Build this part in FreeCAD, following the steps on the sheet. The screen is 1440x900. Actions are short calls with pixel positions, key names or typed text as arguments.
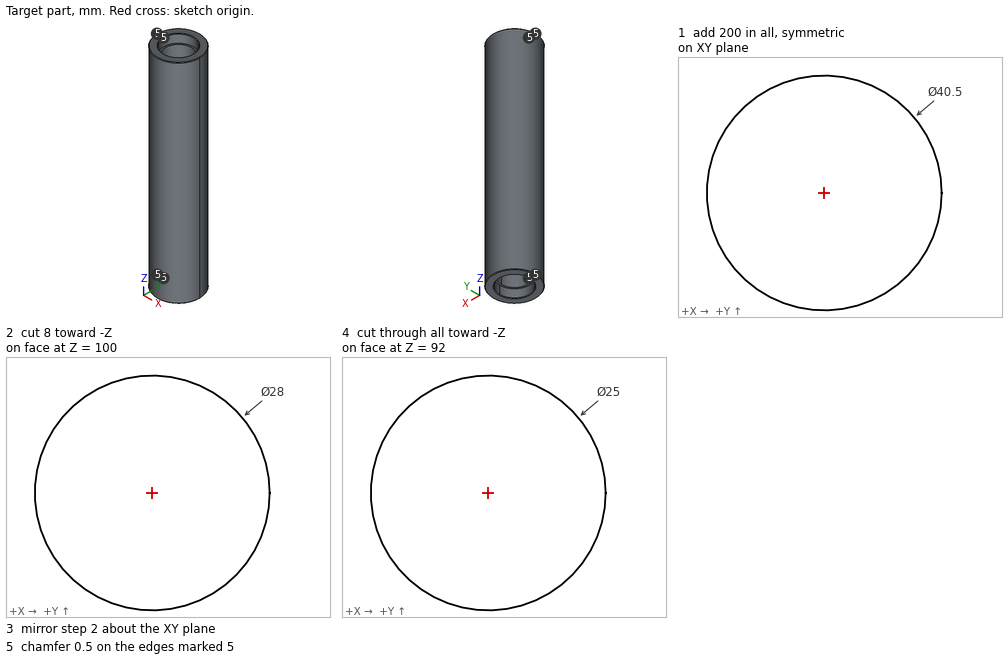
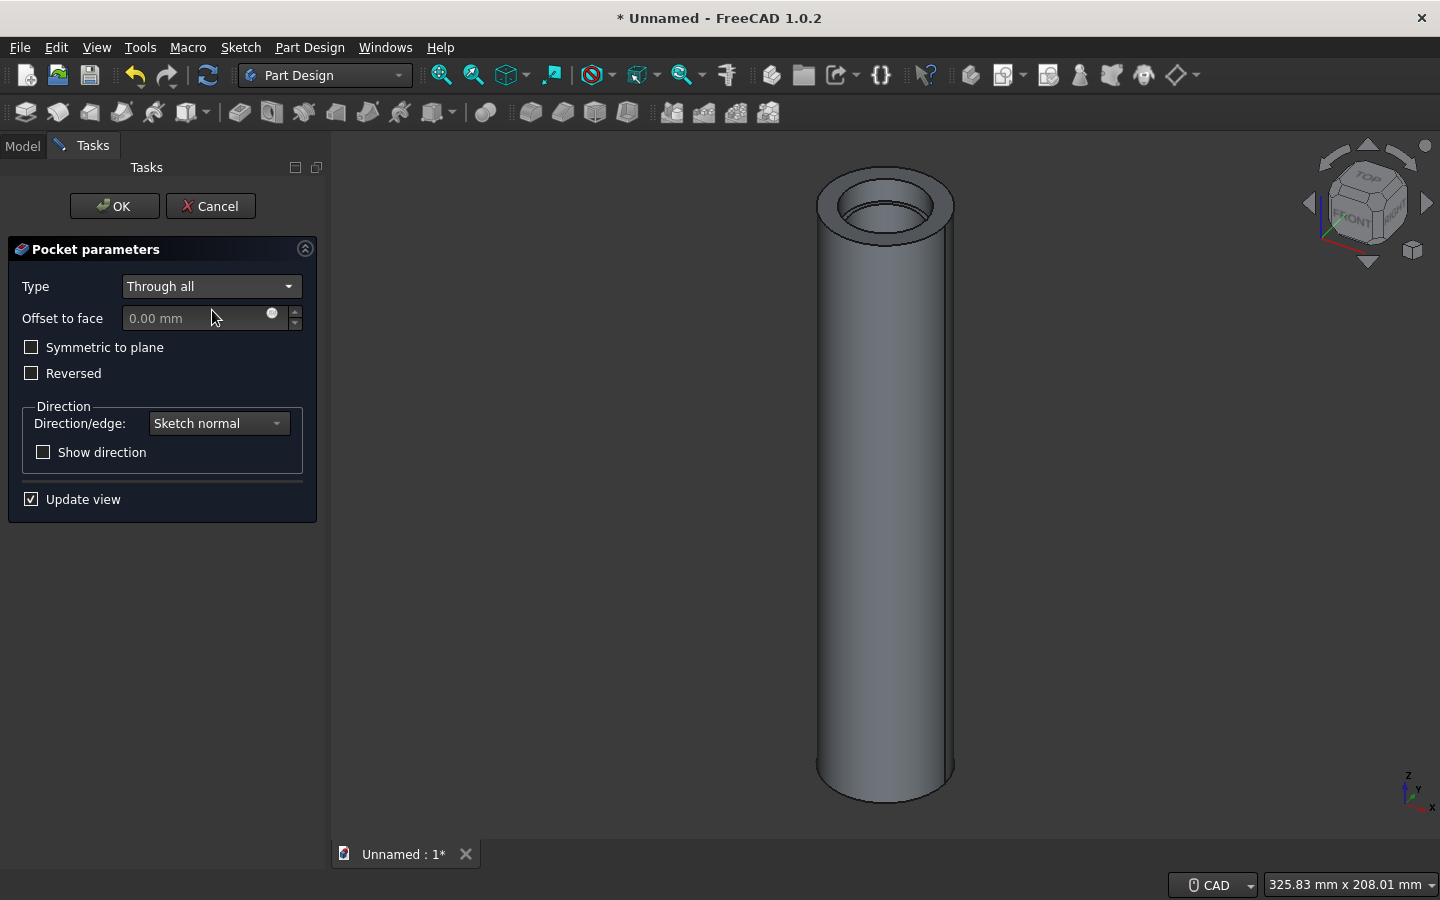
click(115, 206)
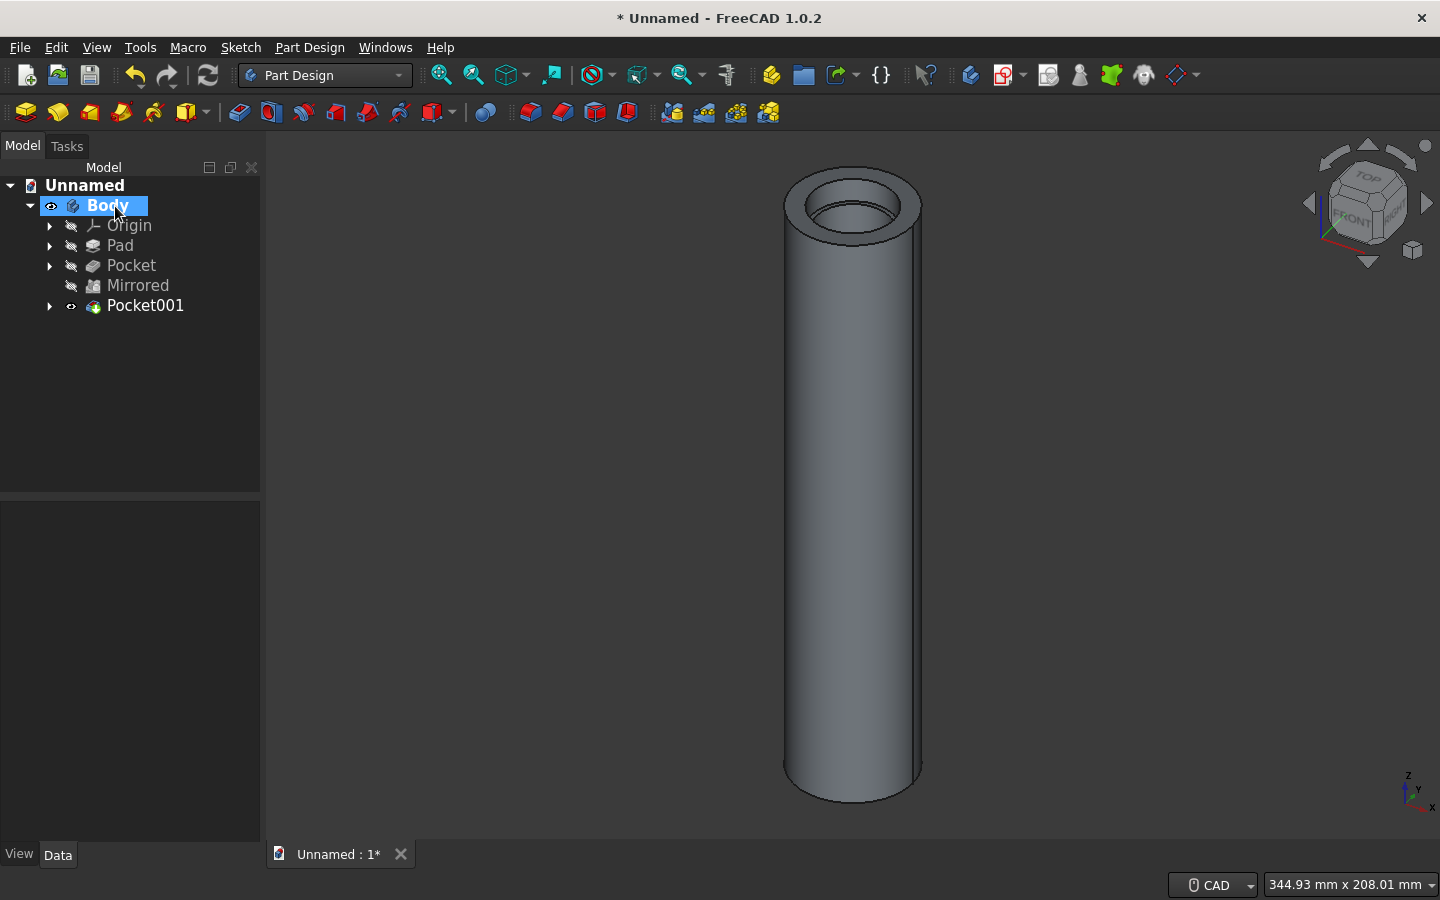
click(784, 209)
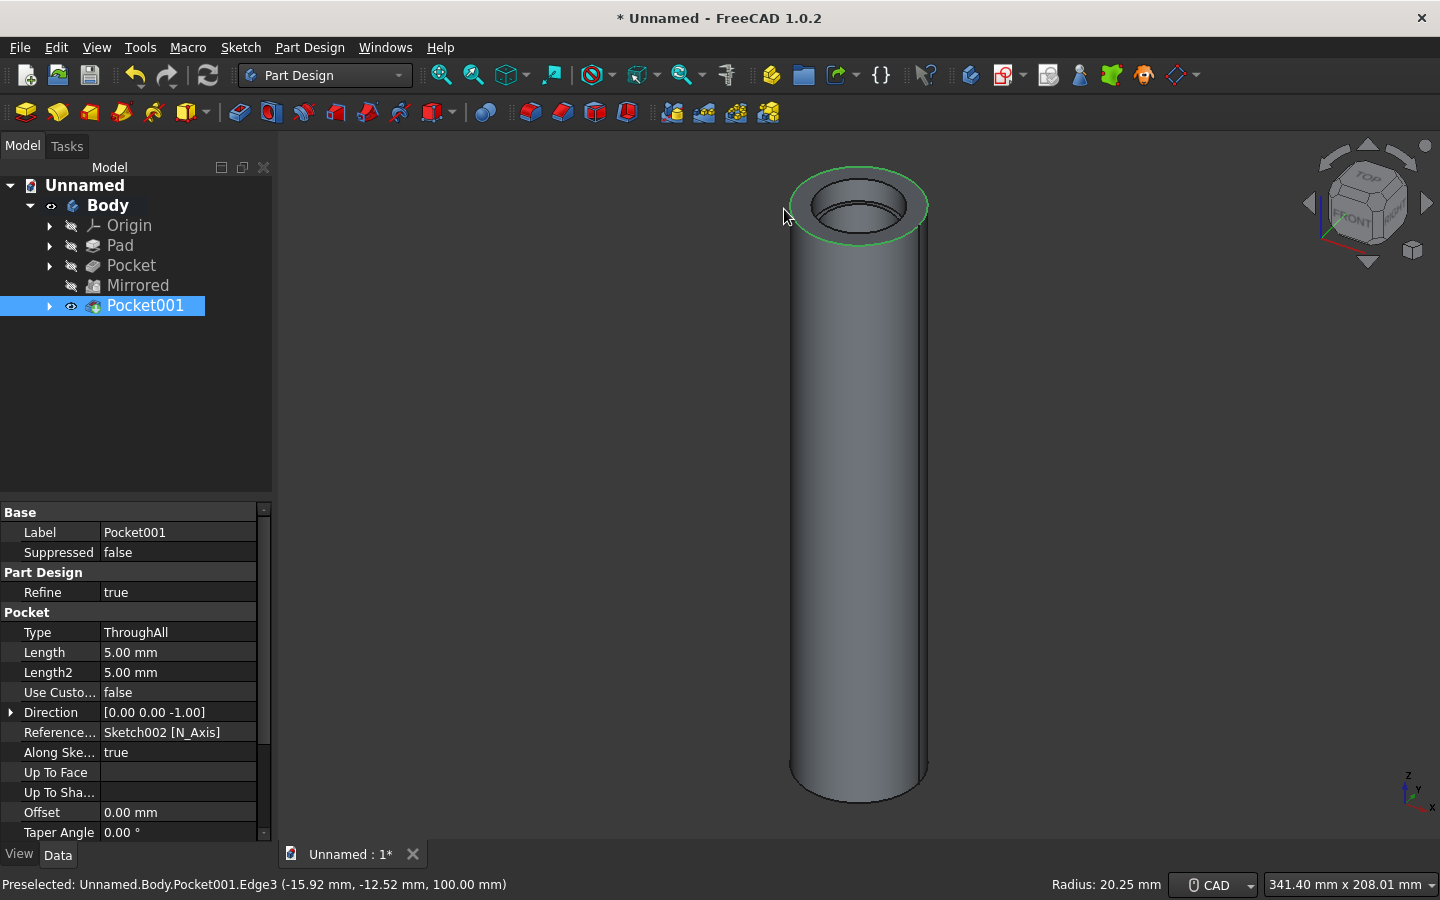
click(818, 191, ctrl)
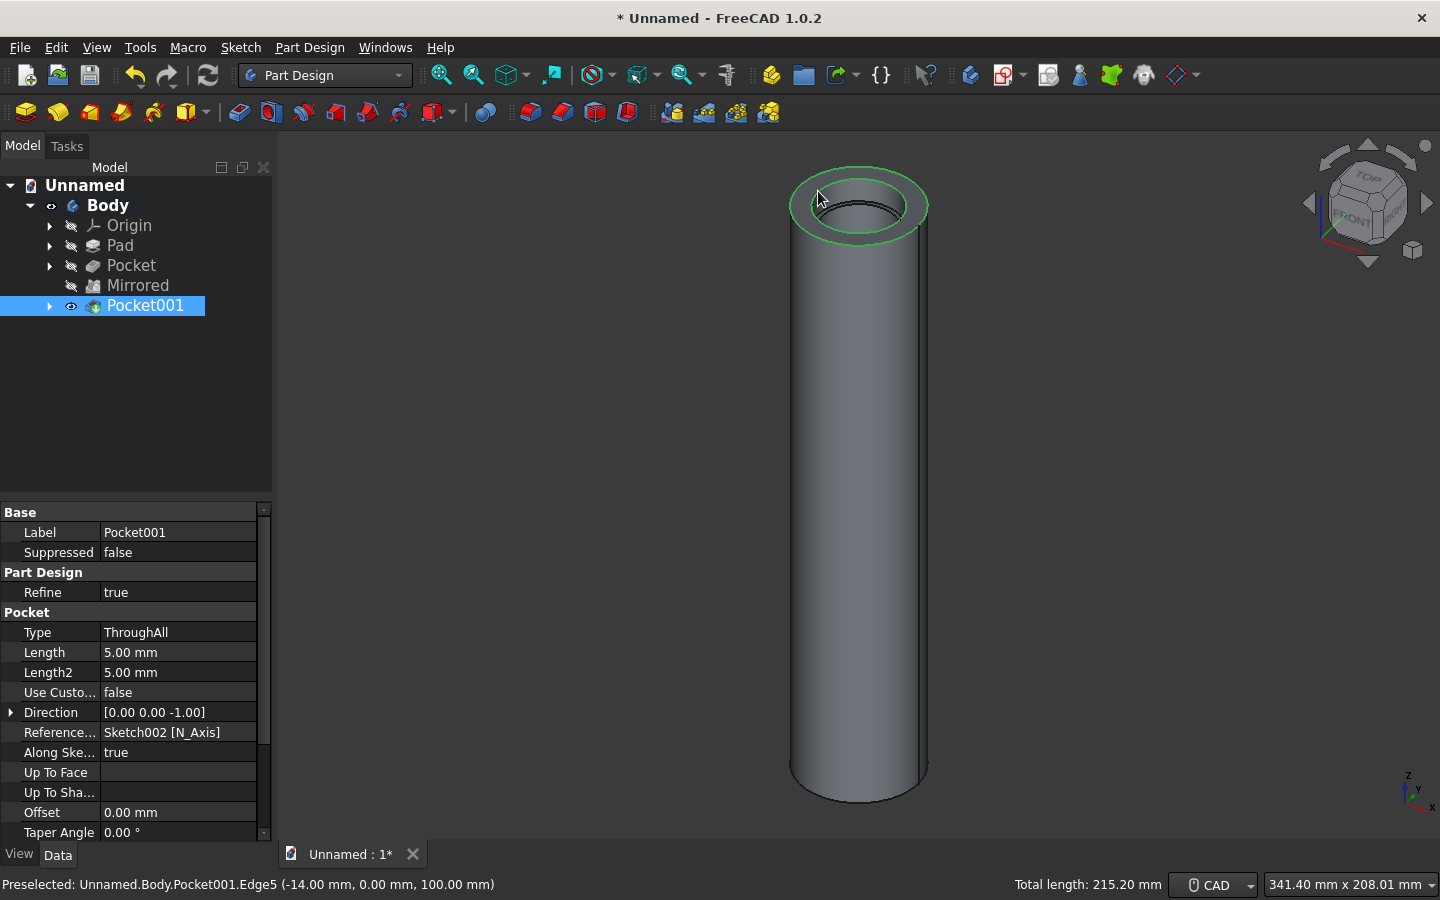
key(0)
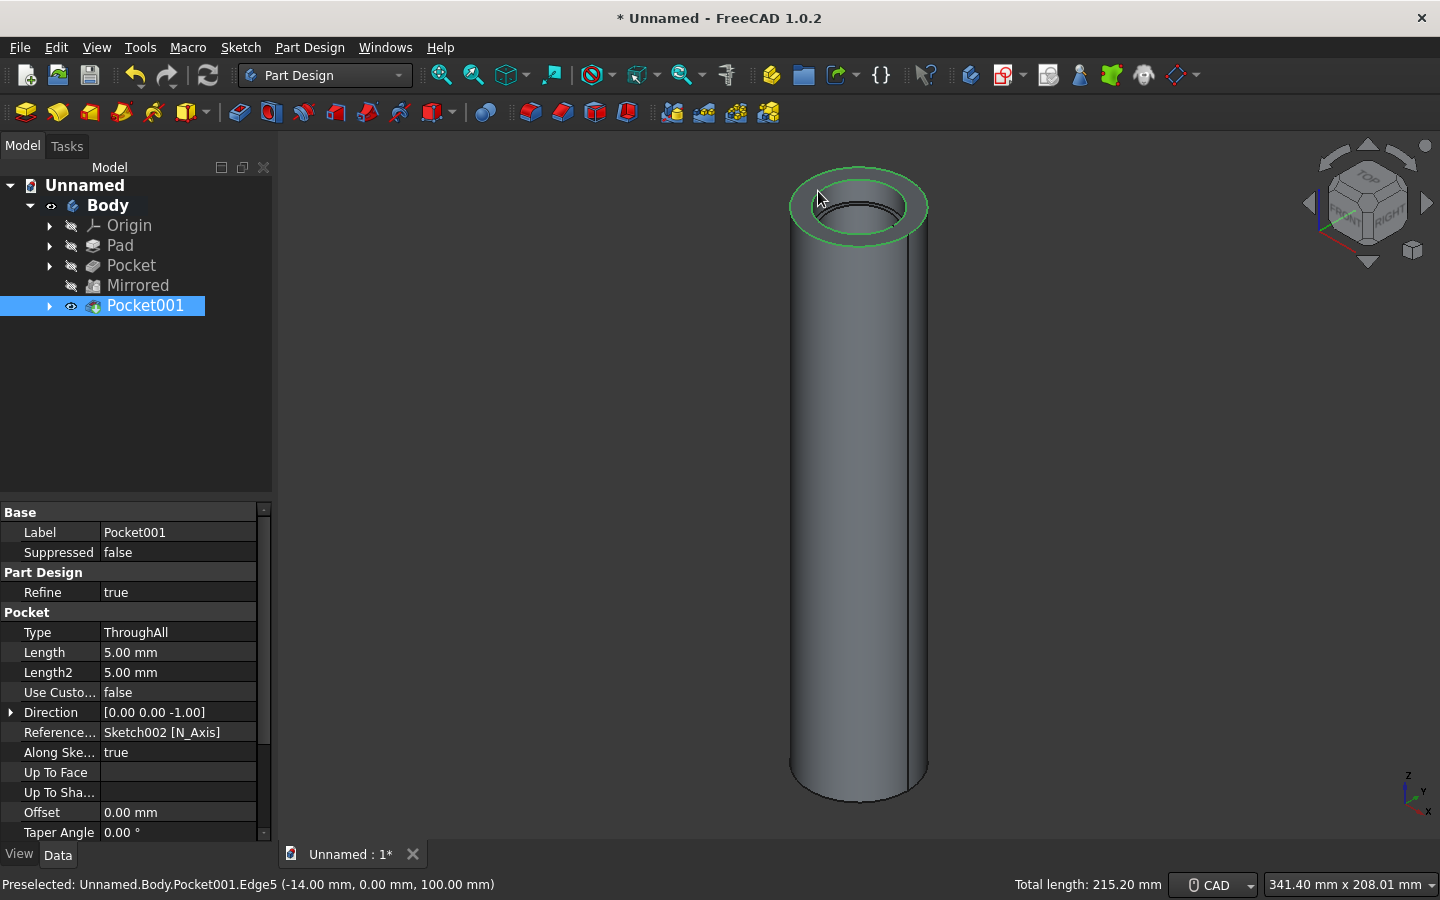
key(2)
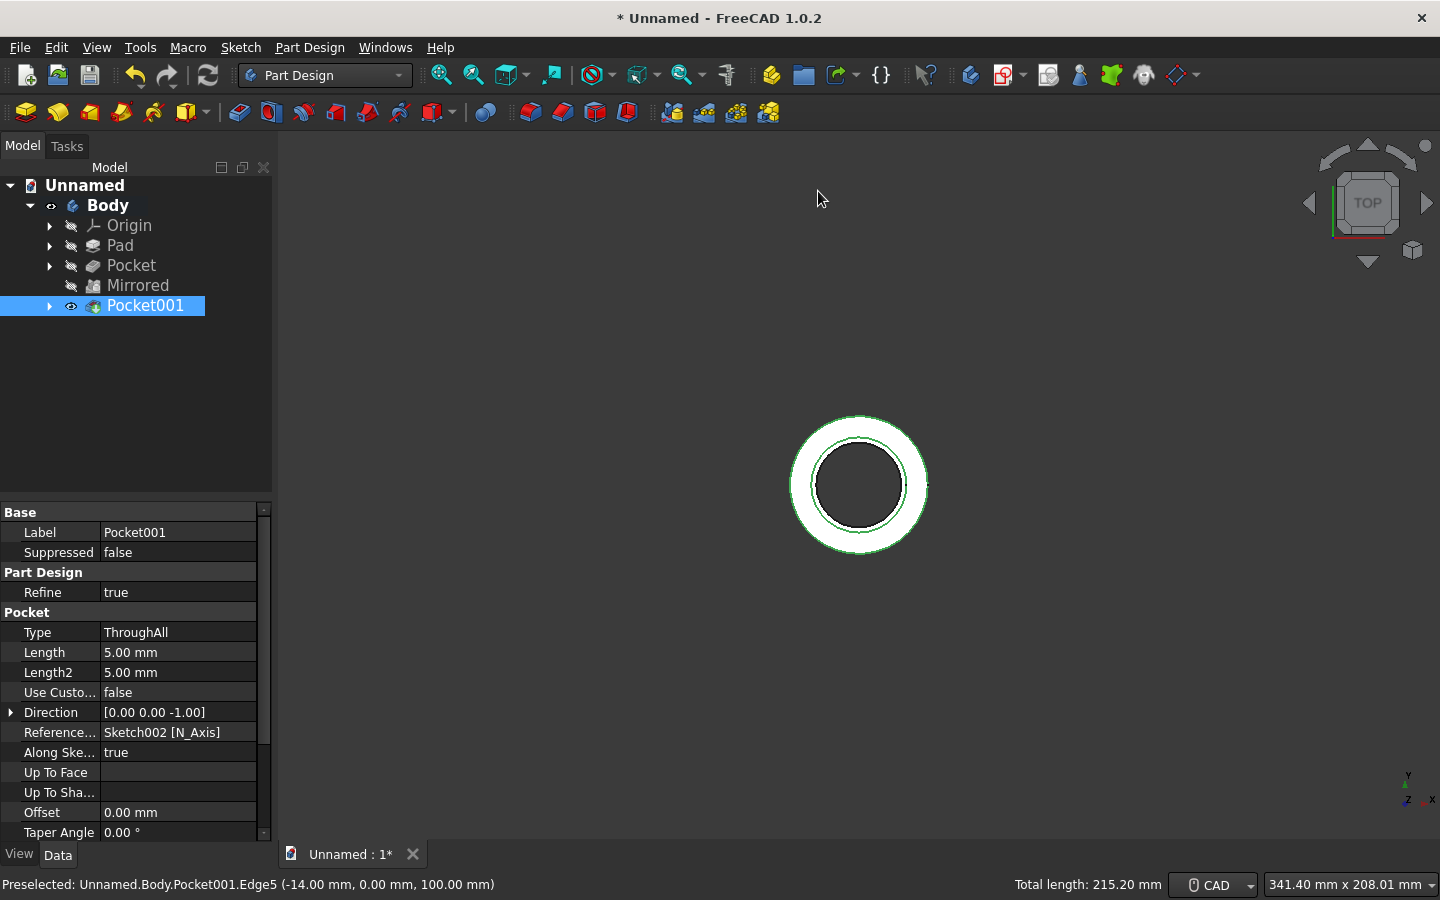
click(442, 76)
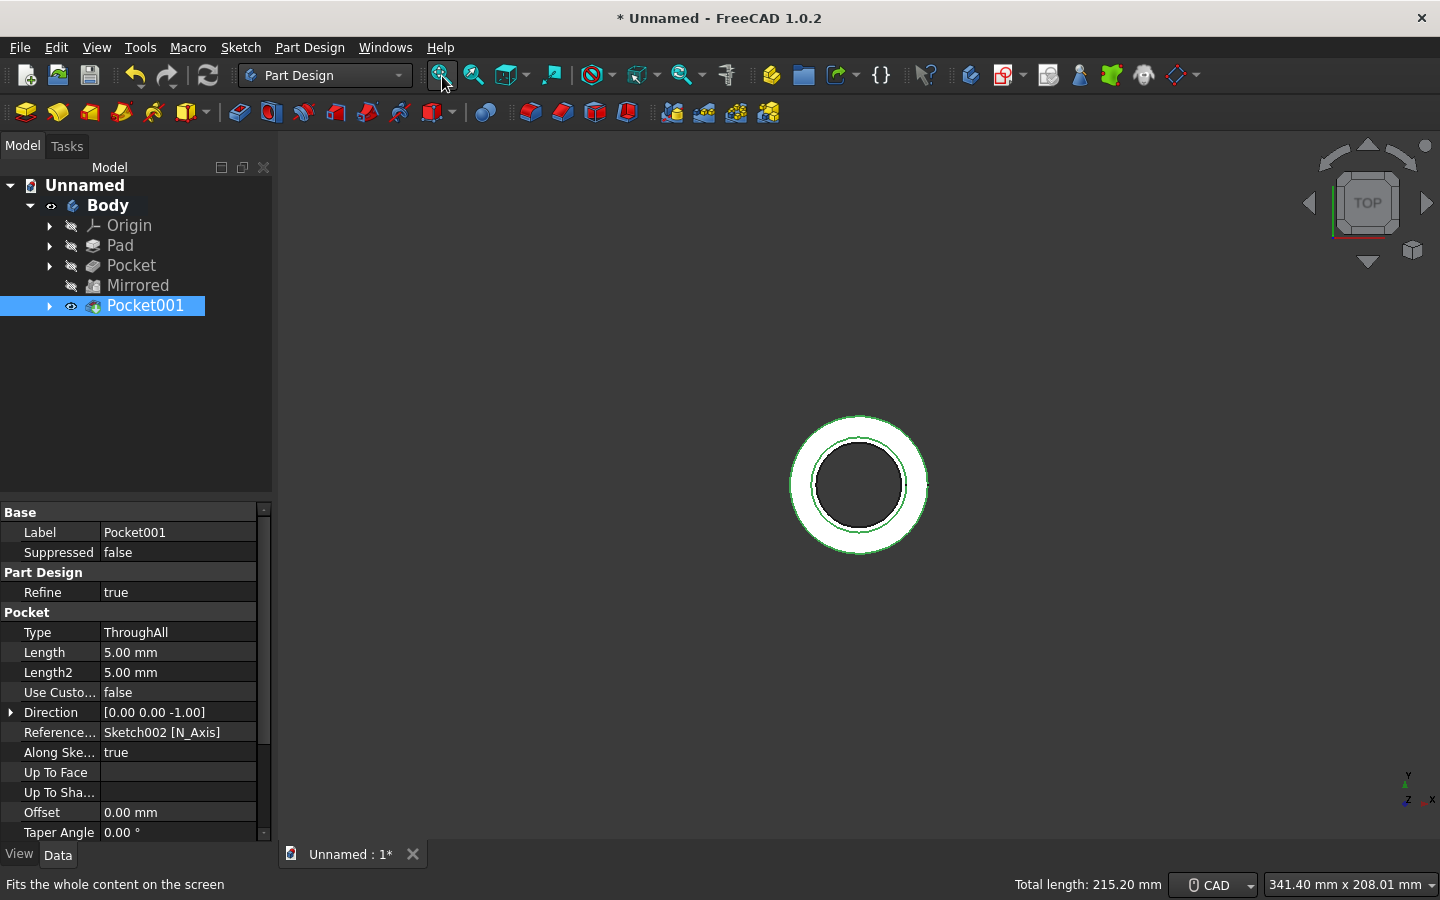
key(1)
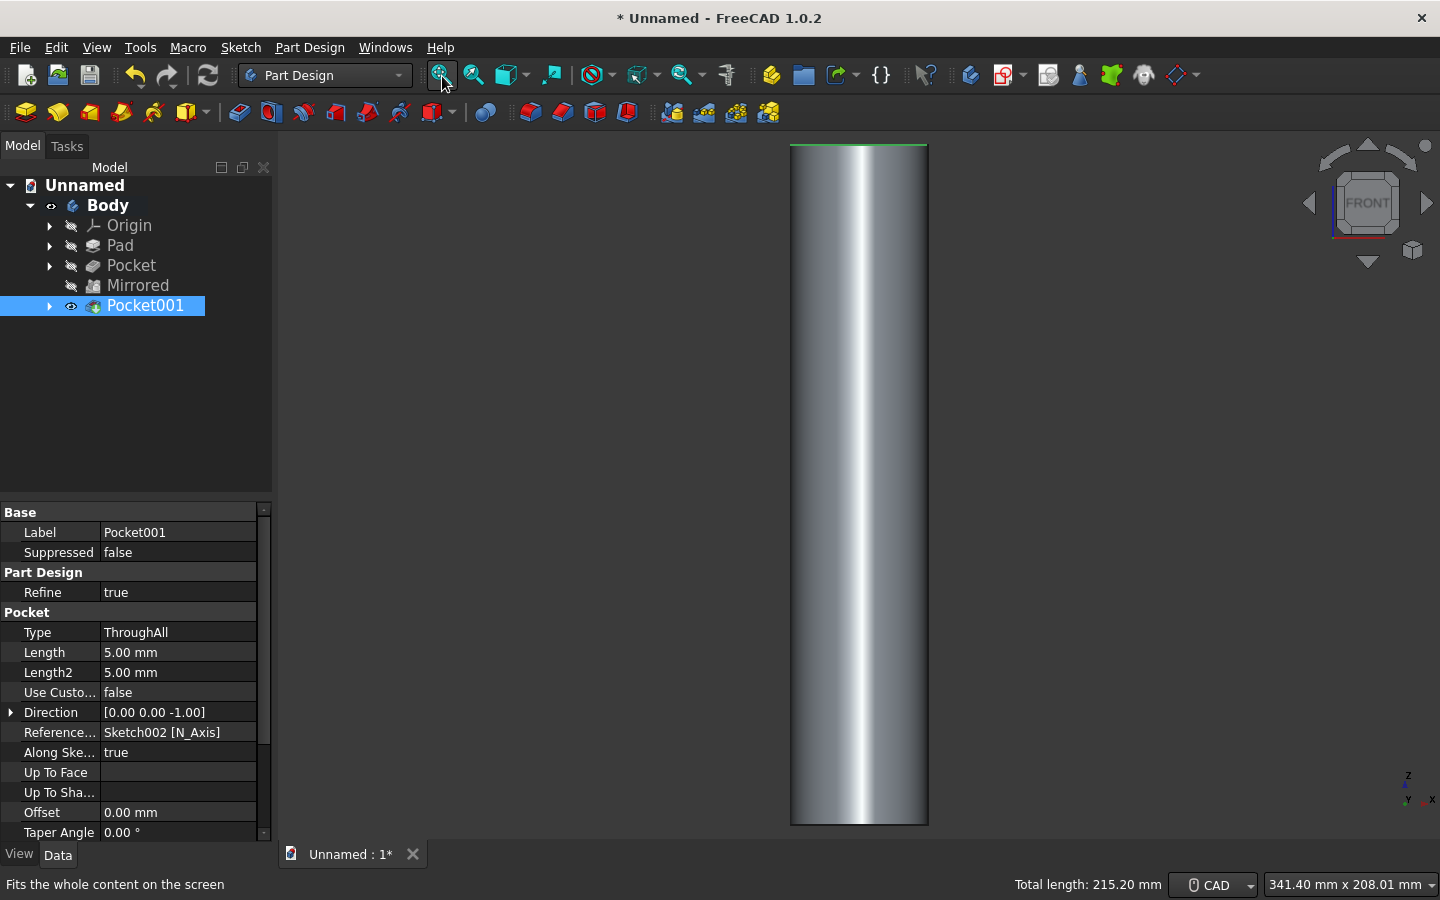
key(3)